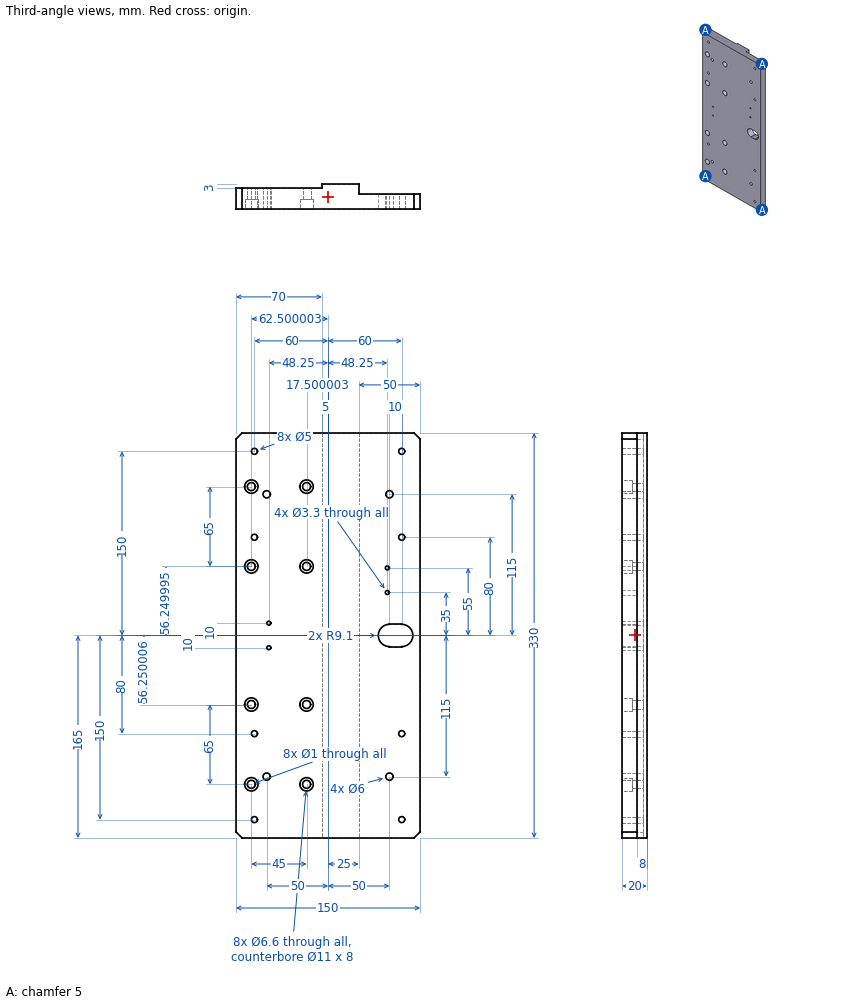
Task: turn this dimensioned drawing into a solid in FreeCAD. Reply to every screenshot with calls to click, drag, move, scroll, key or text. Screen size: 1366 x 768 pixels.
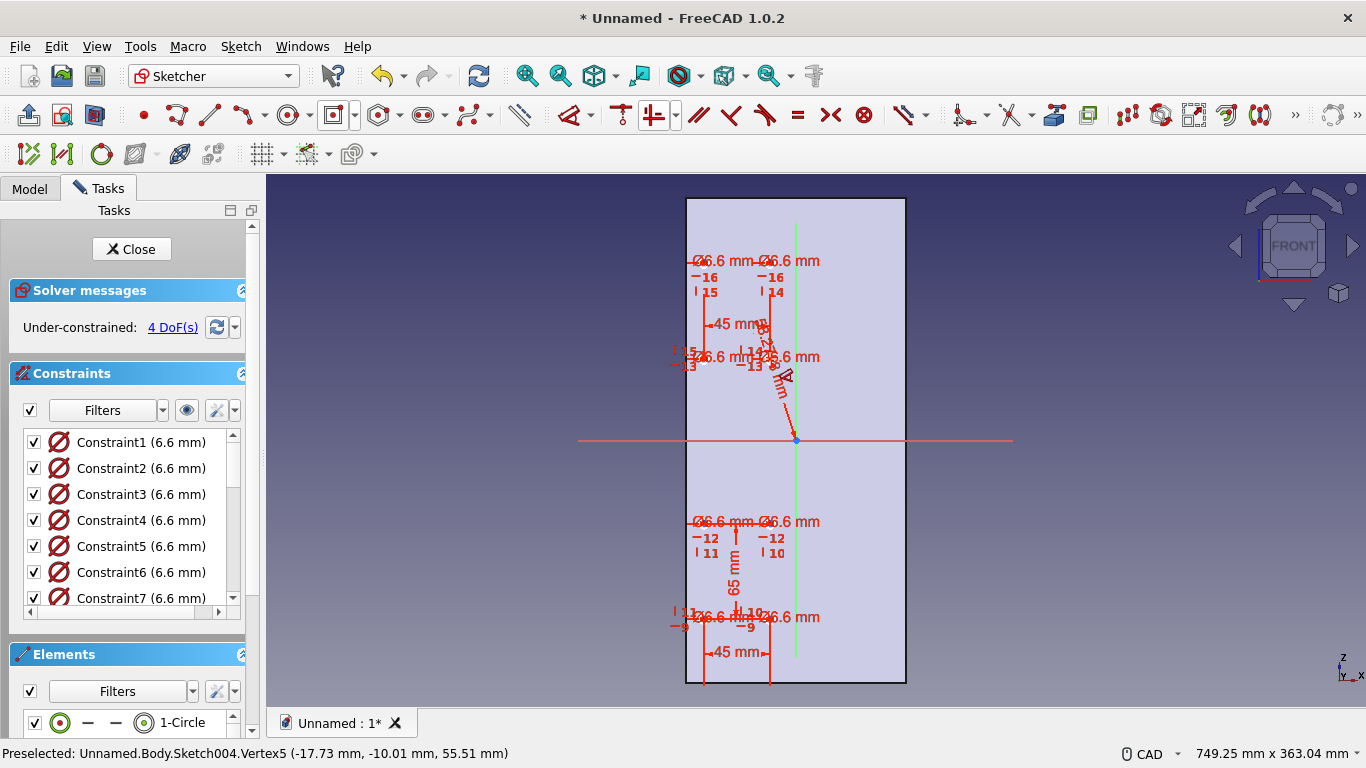
click(770, 263)
click(736, 289)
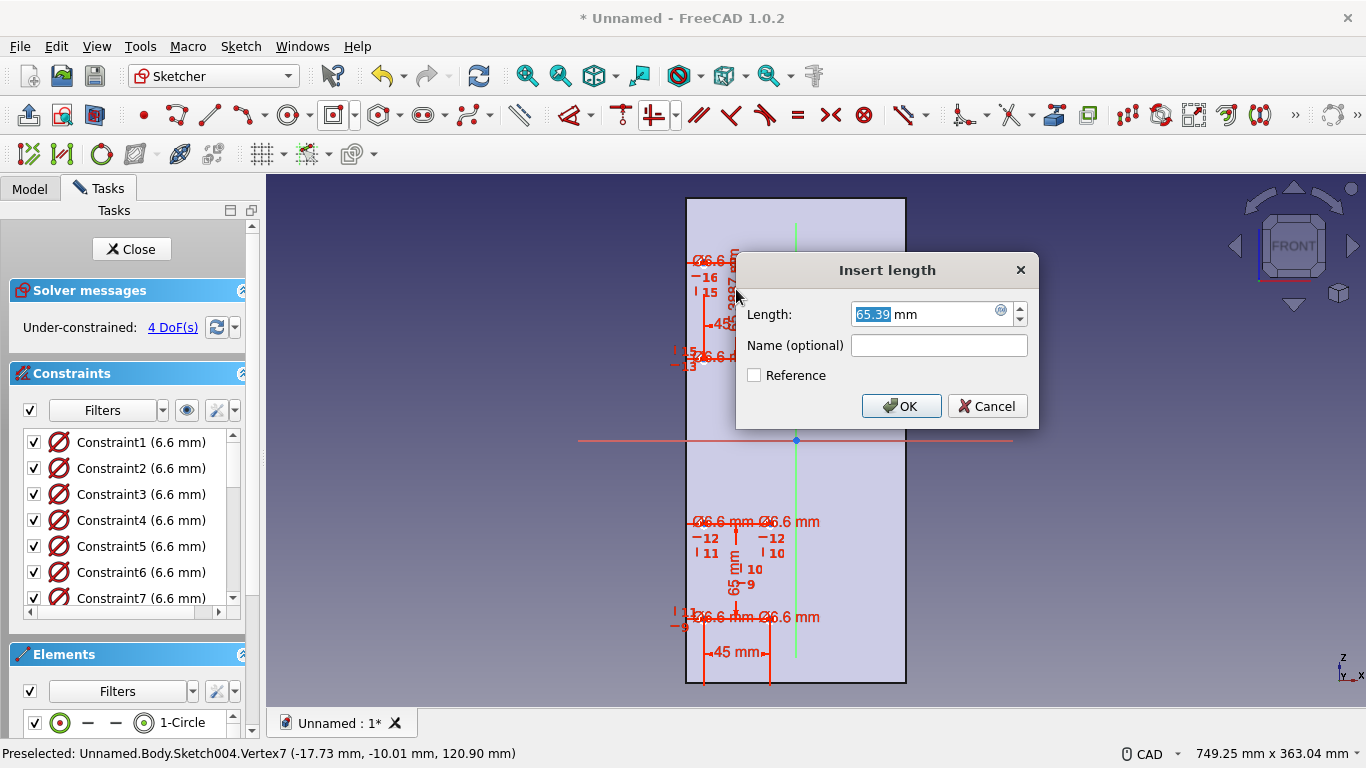
text(65)
key(Return)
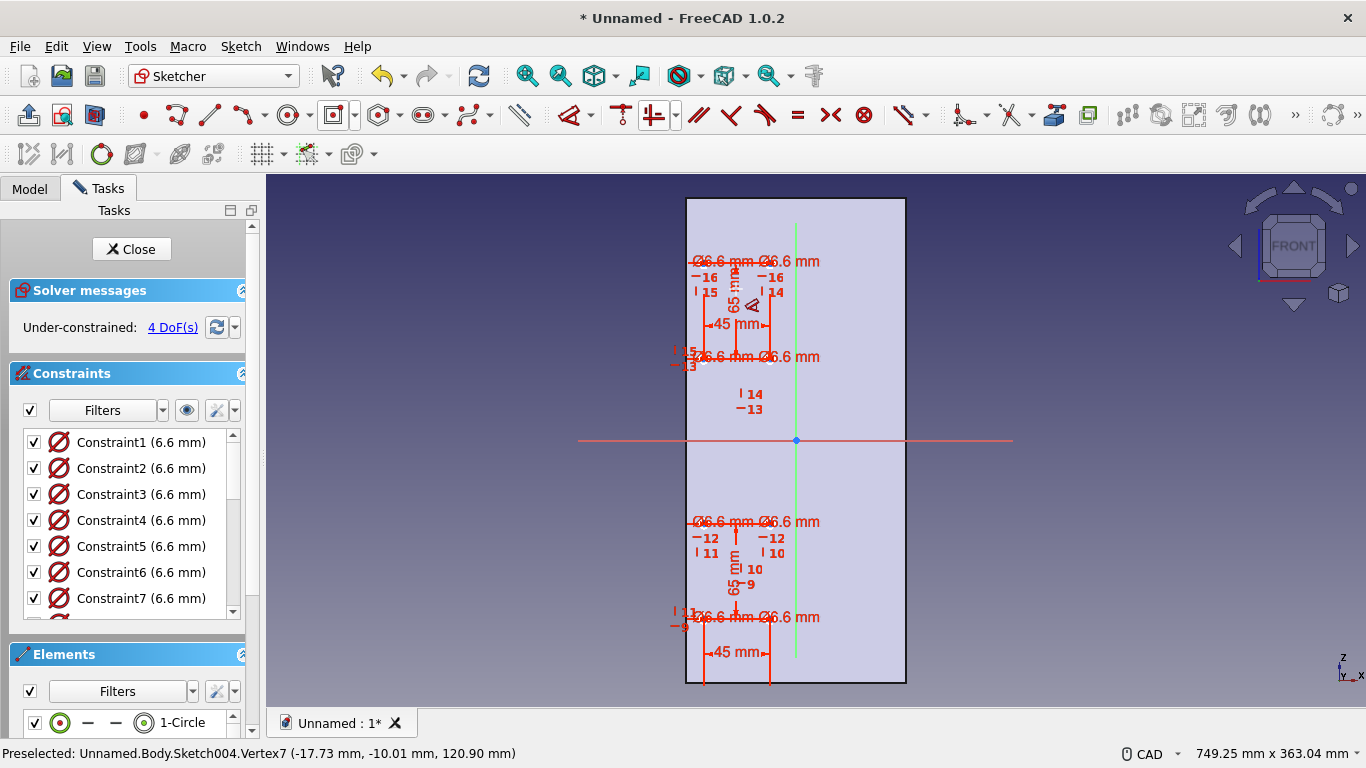
scroll(770, 619, up, 3)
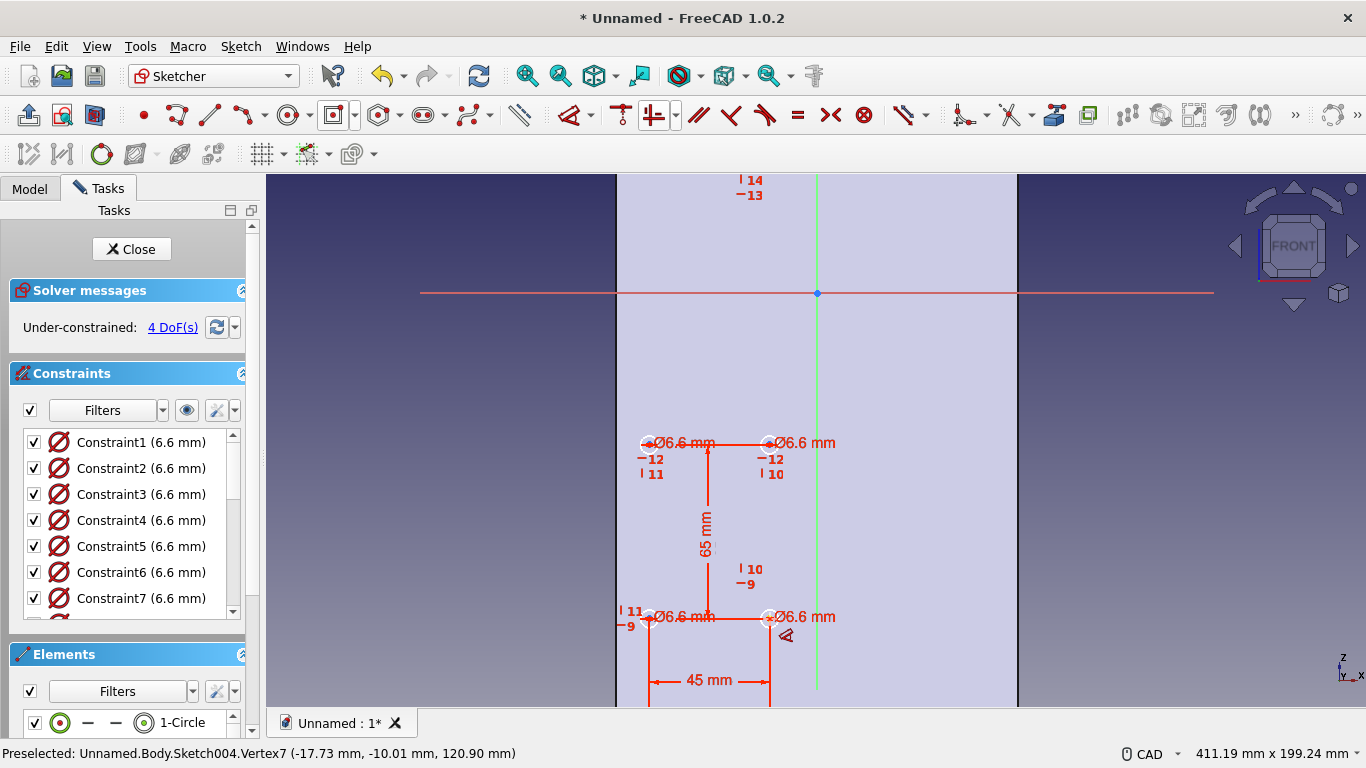
click(770, 619)
click(793, 653)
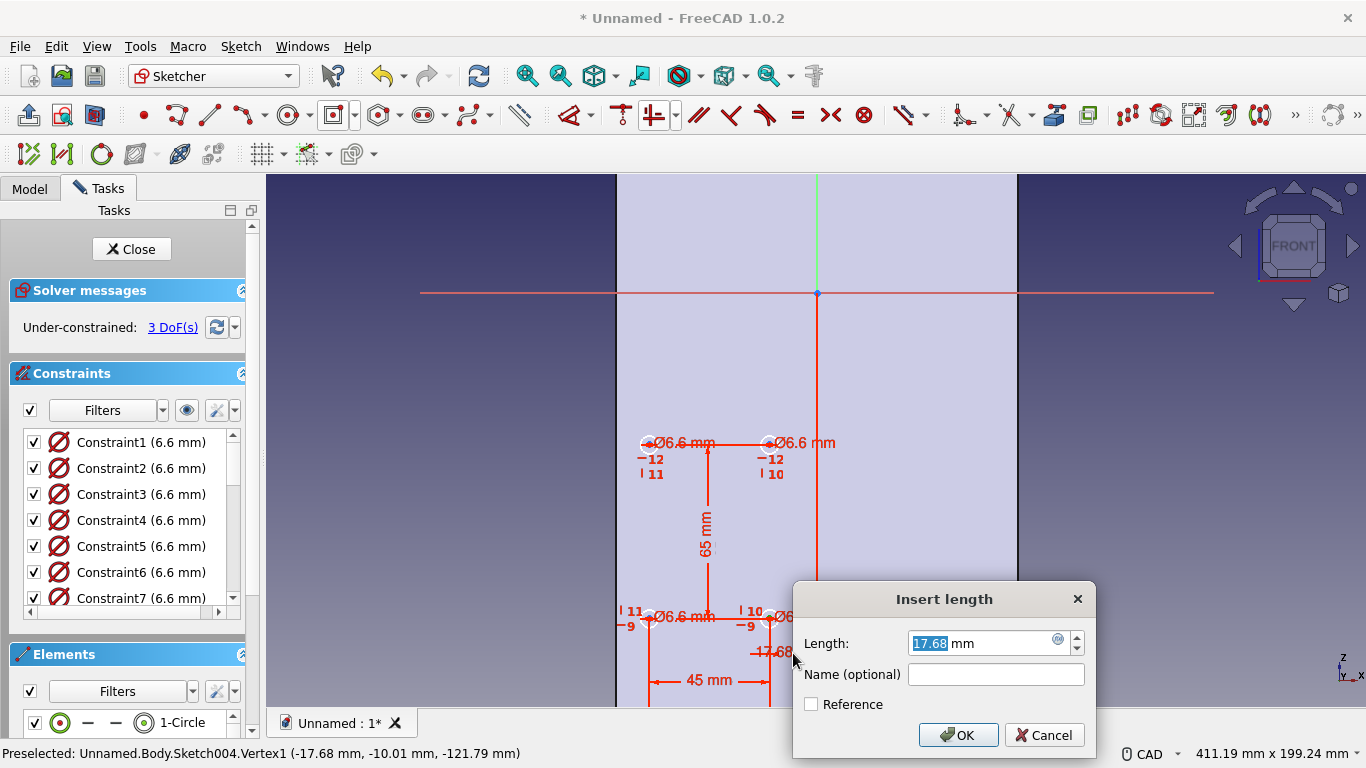
text(17.500006)
key(Return)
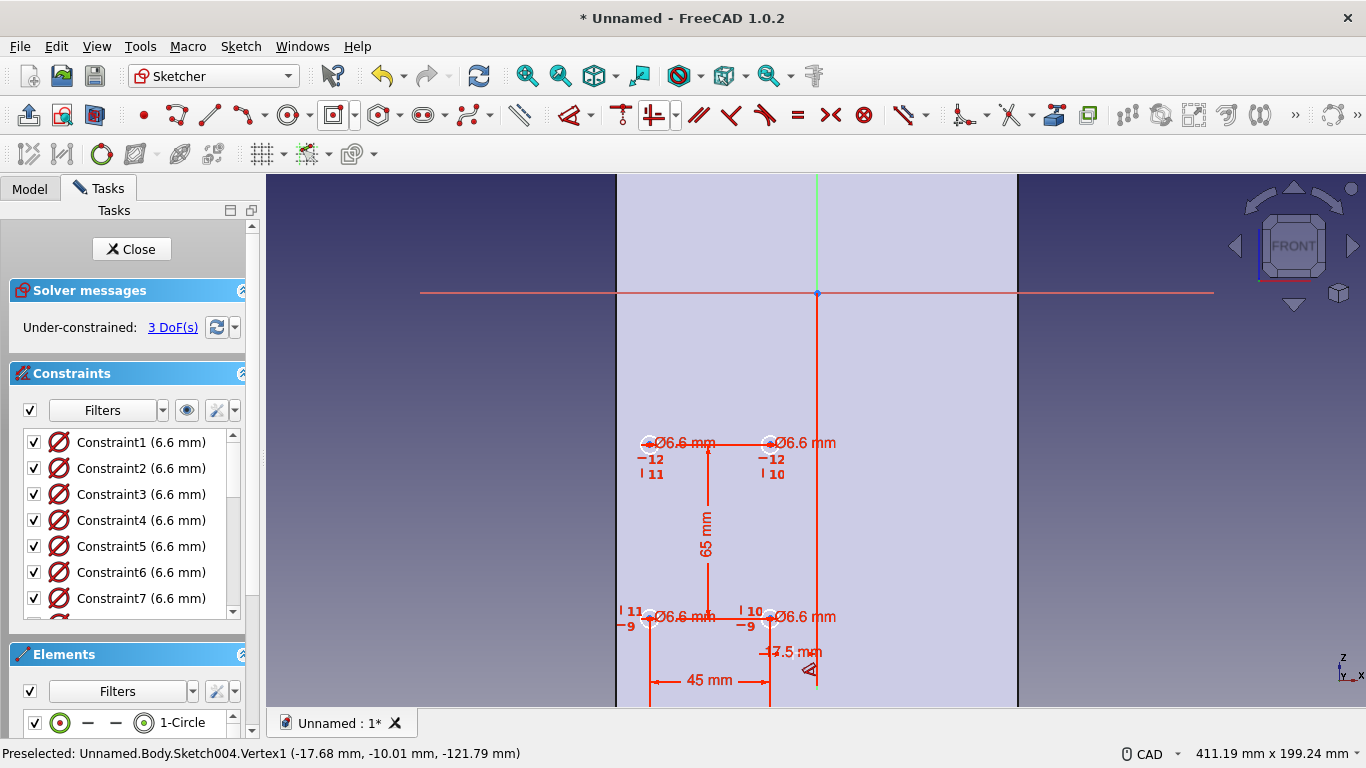
click(770, 445)
click(851, 369)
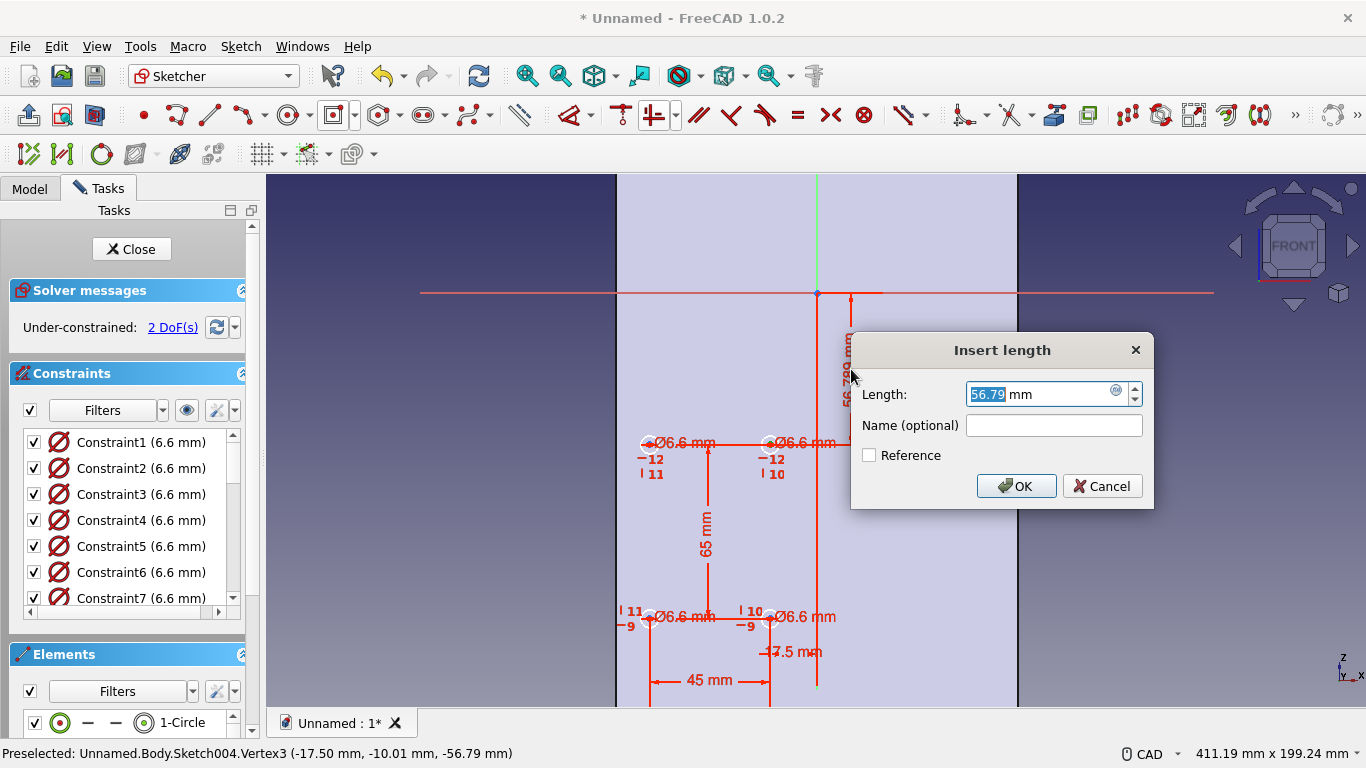
text(56.250006)
key(Return)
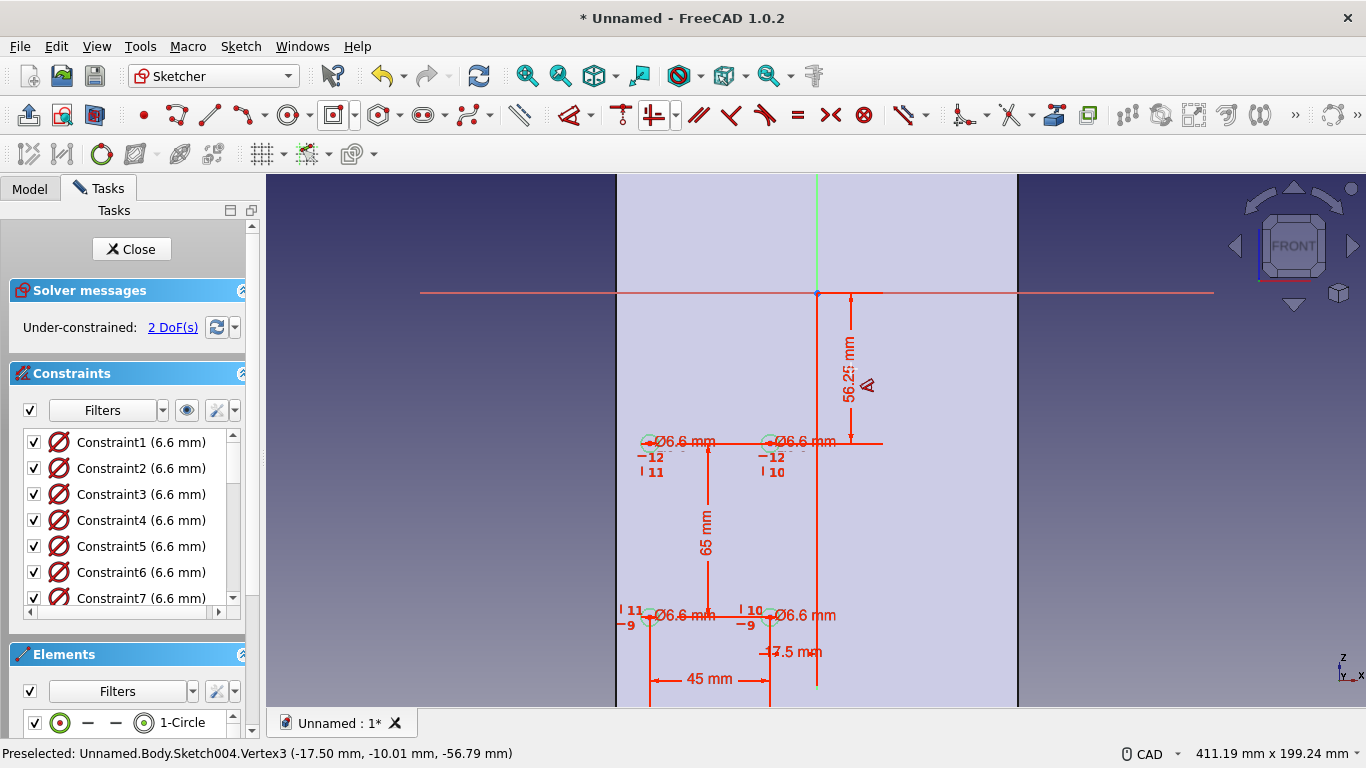
scroll(770, 620, down, 3)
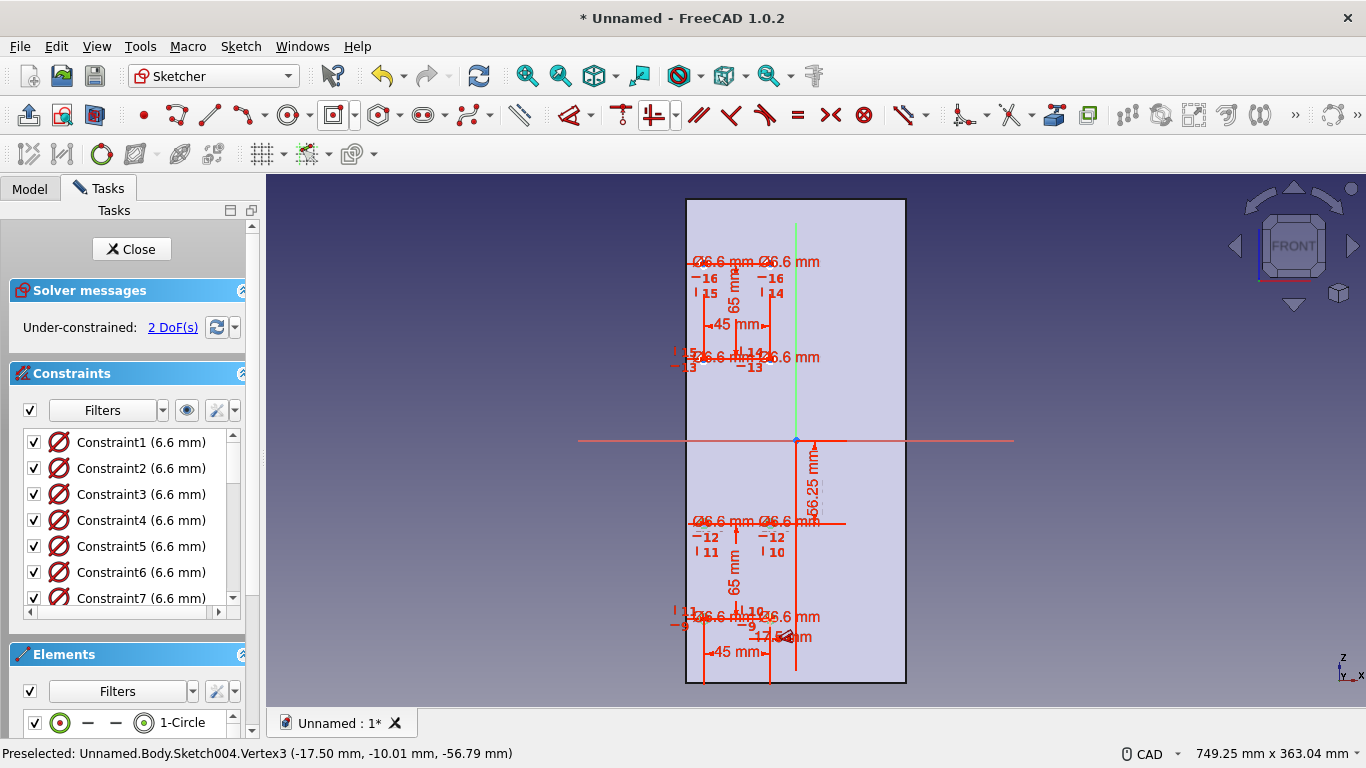
scroll(770, 359, up, 3)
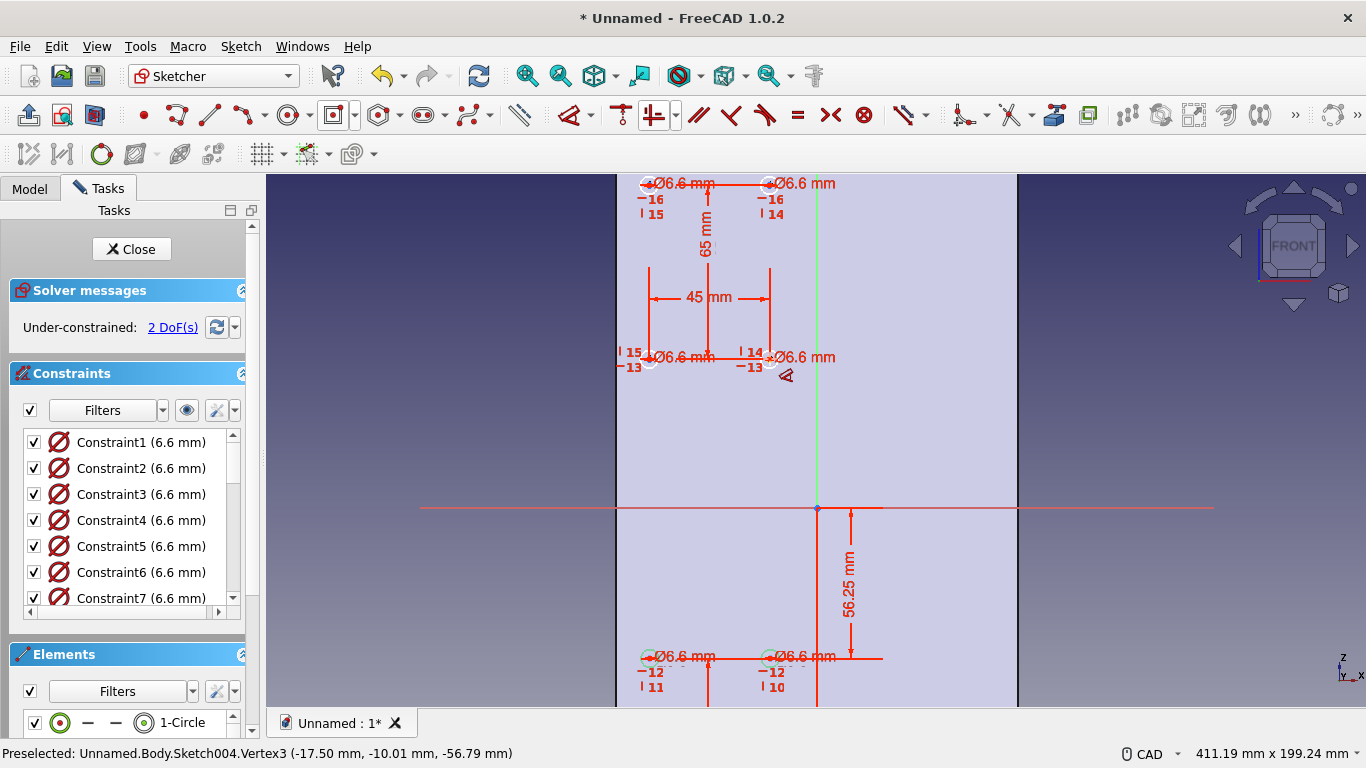
click(770, 359)
click(793, 325)